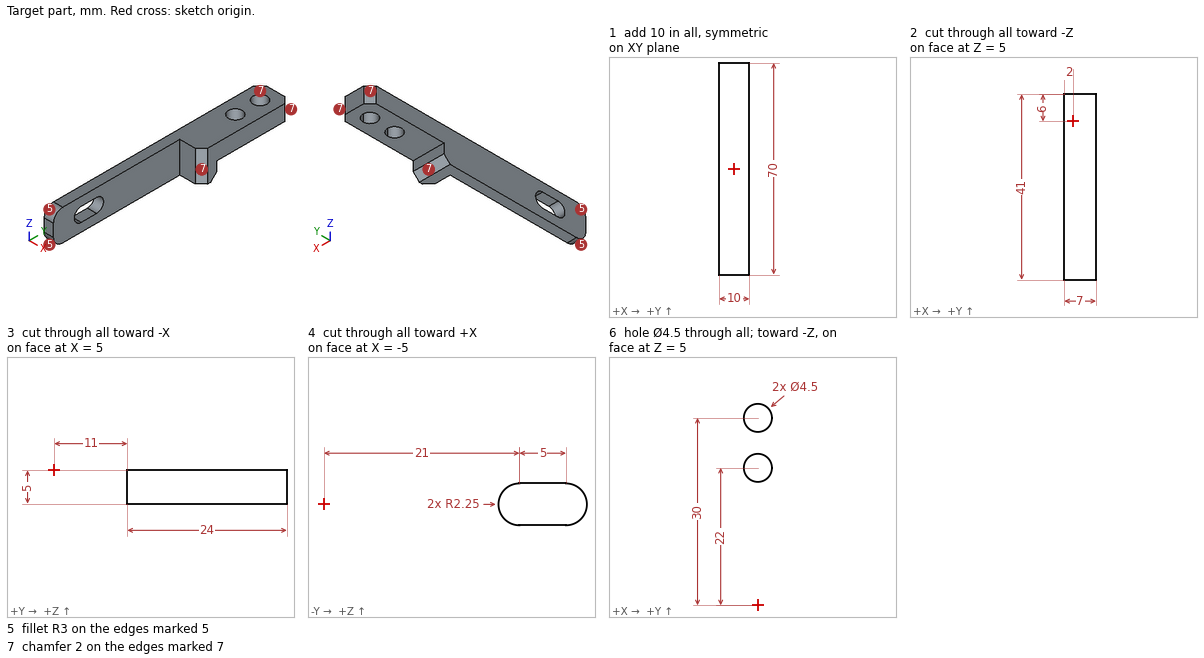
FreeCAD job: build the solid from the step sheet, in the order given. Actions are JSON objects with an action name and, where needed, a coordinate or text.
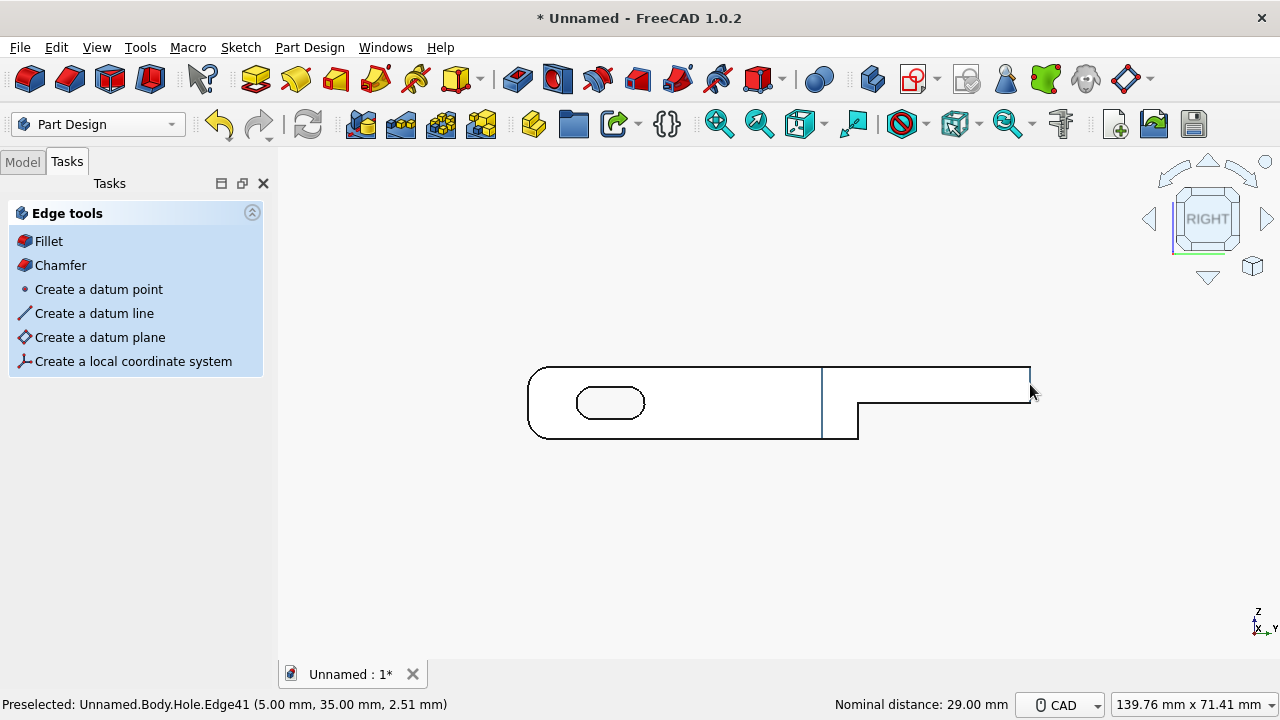
{"action": "key", "text": "5"}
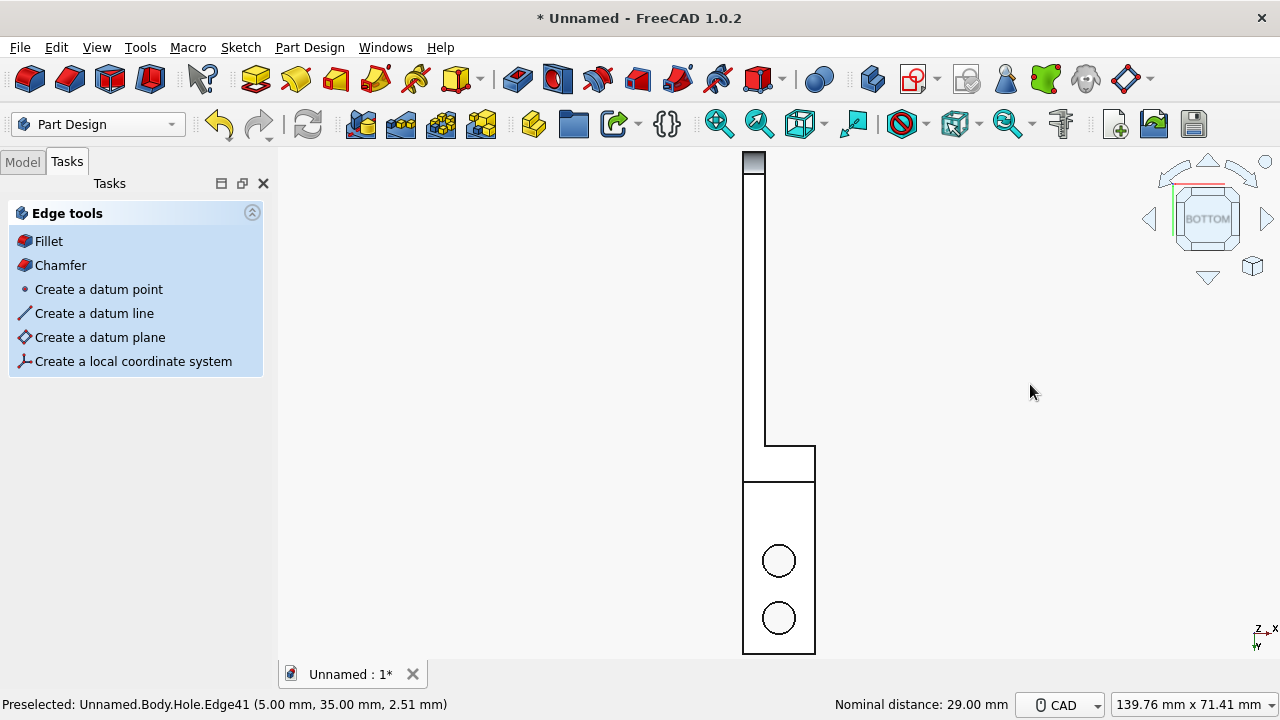
{"action": "left_click", "coordinate": [779, 481], "text": "ctrl"}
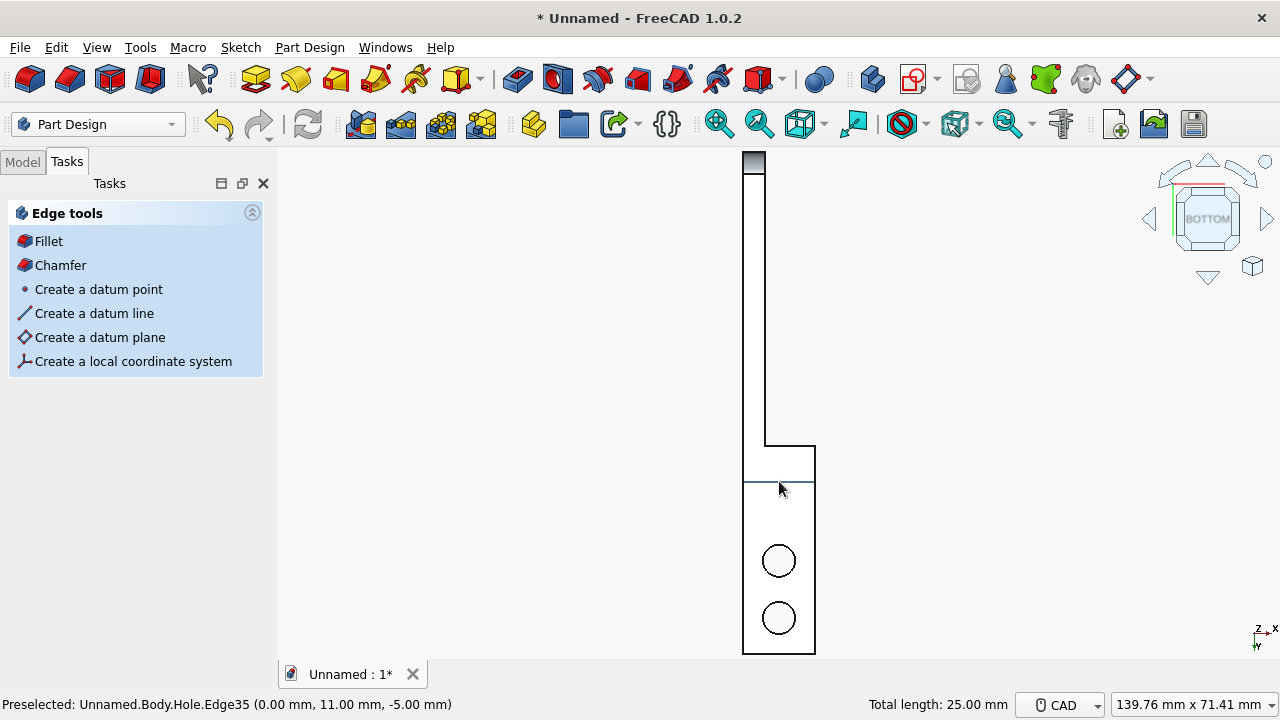
{"action": "key", "text": "4"}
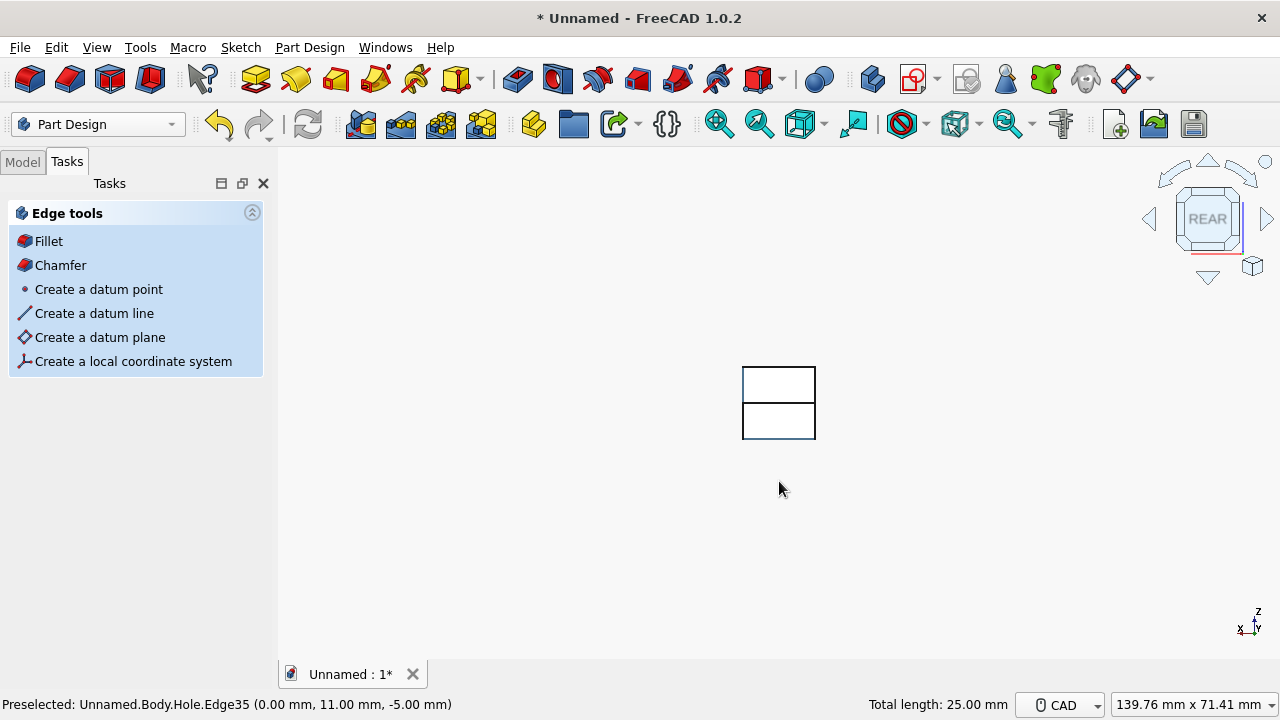
{"action": "key", "text": "v f"}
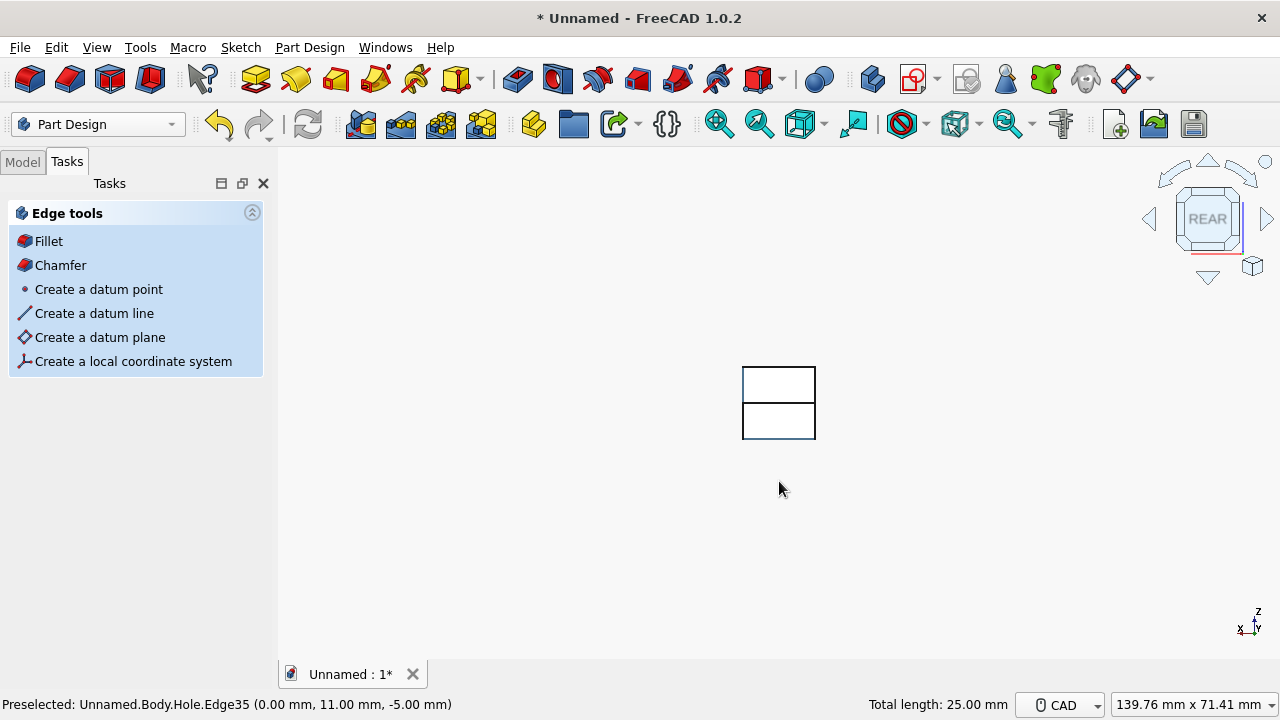
{"action": "left_click", "coordinate": [815, 384], "text": "ctrl"}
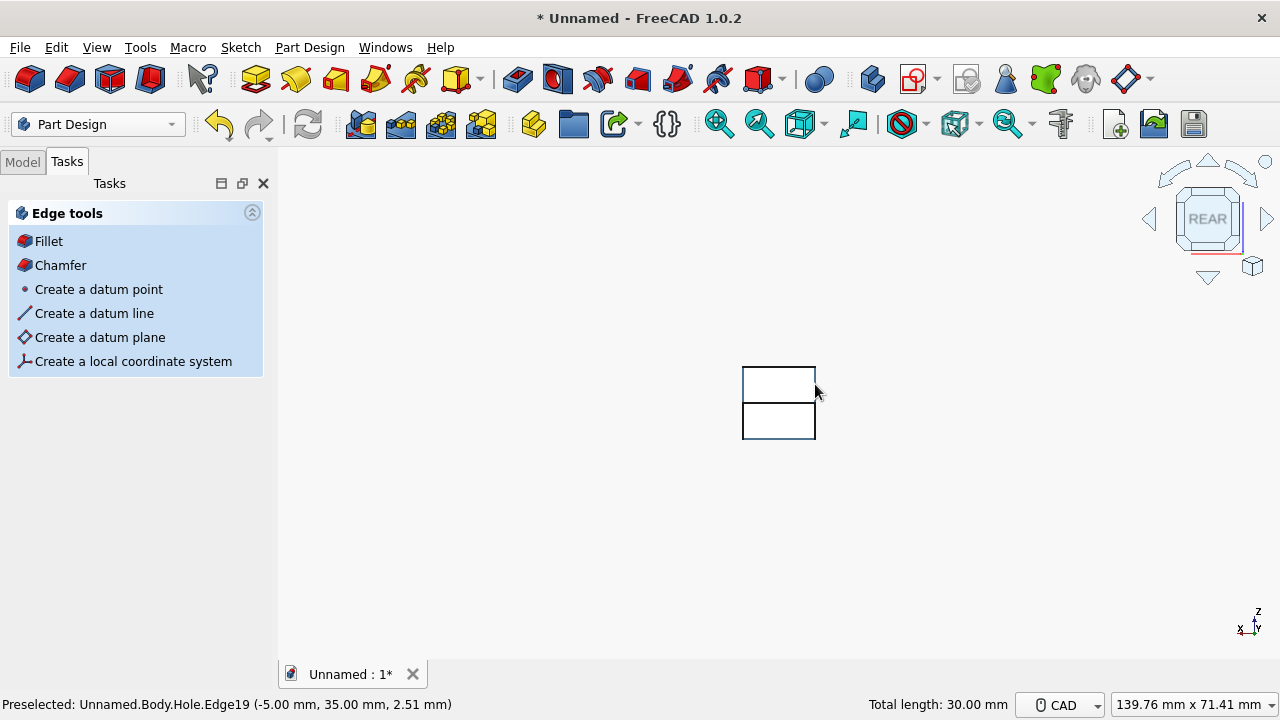
{"action": "left_click", "coordinate": [70, 80]}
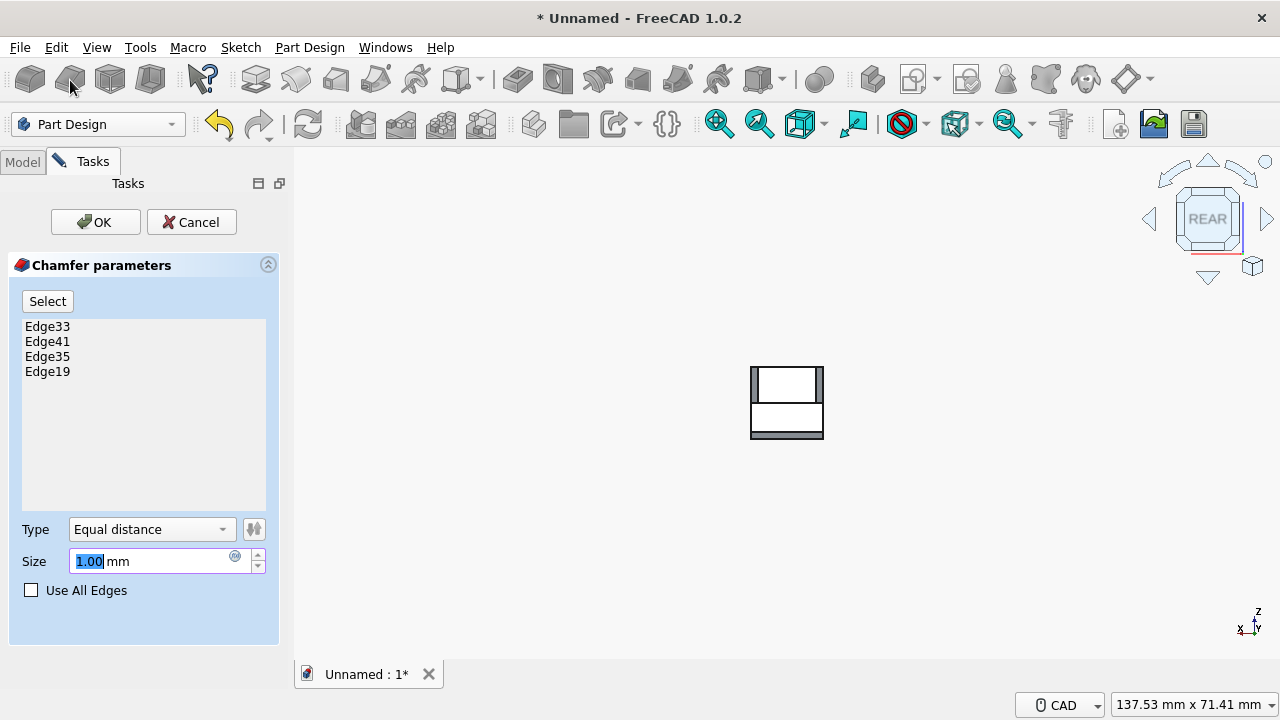
{"action": "type", "text": "2"}
{"action": "key", "text": "Tab"}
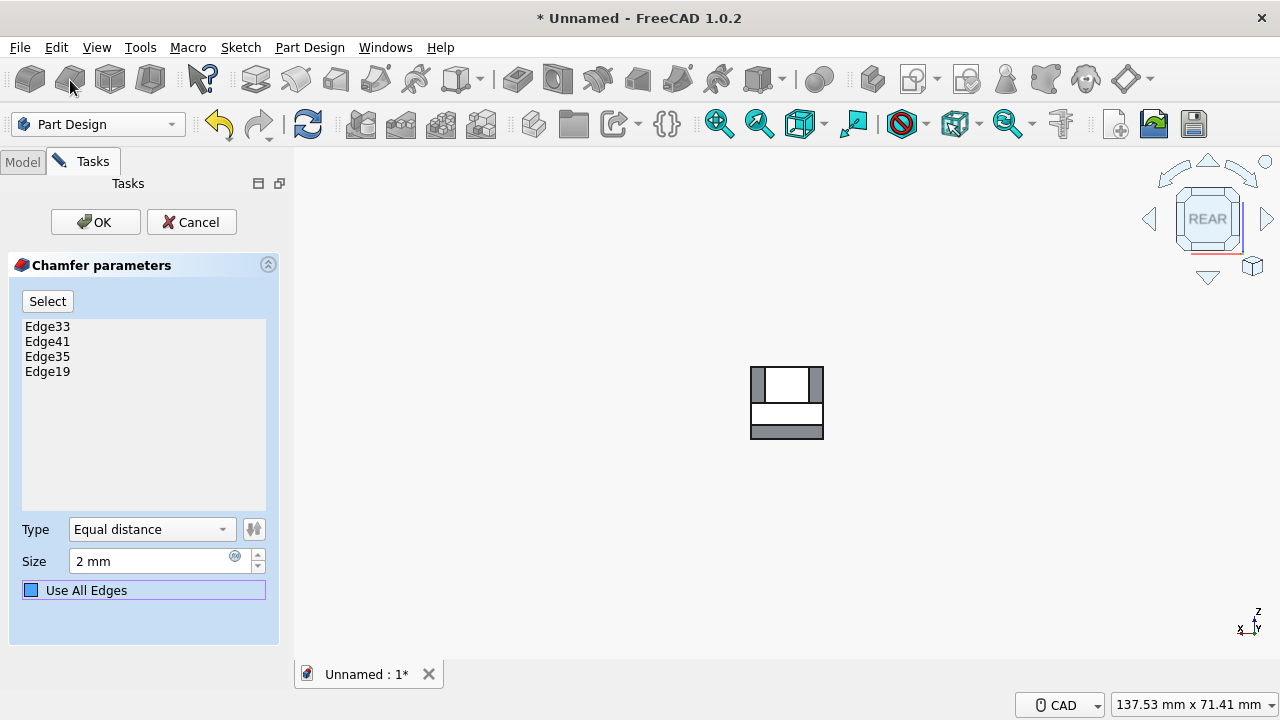
{"action": "left_click", "coordinate": [96, 222]}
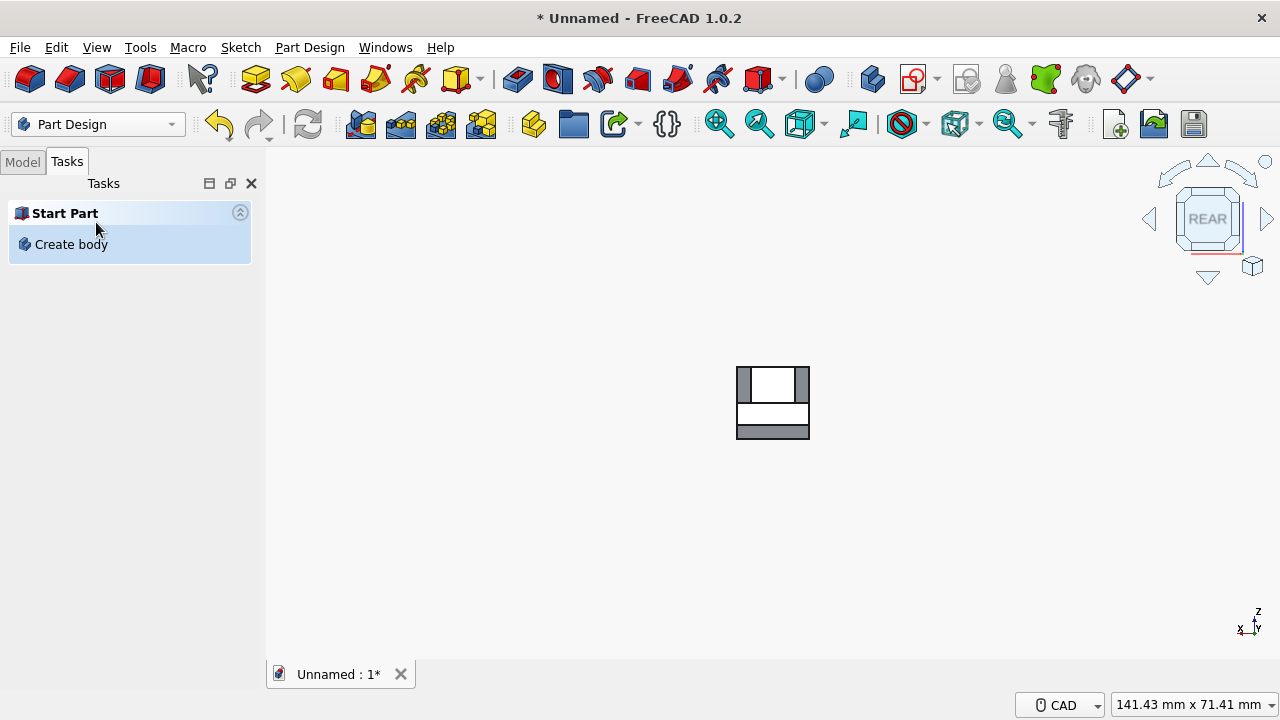
{"action": "key", "text": "0"}